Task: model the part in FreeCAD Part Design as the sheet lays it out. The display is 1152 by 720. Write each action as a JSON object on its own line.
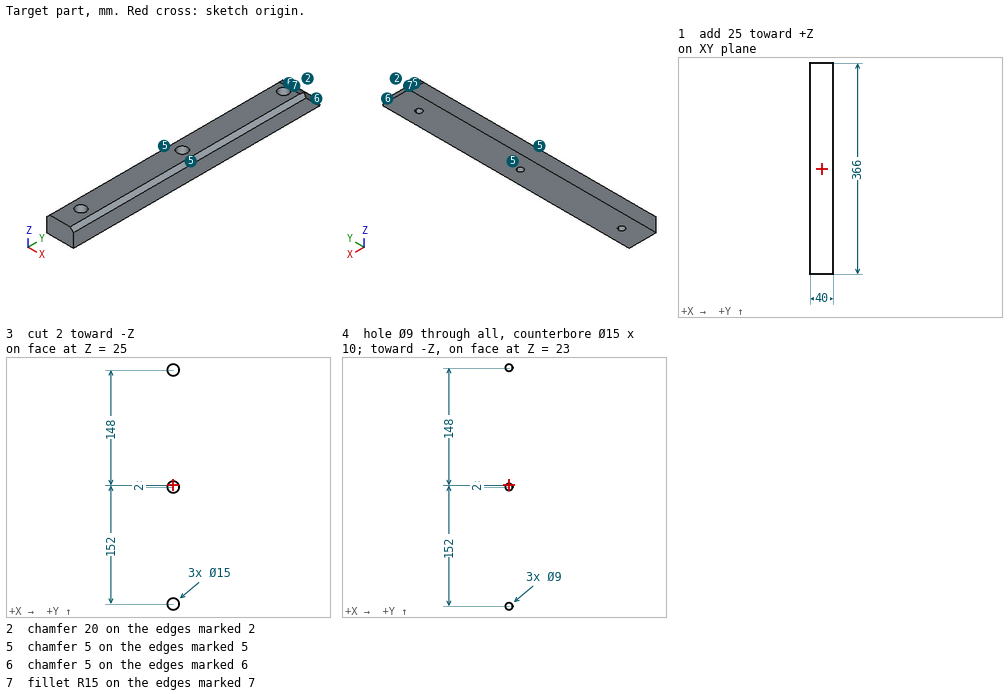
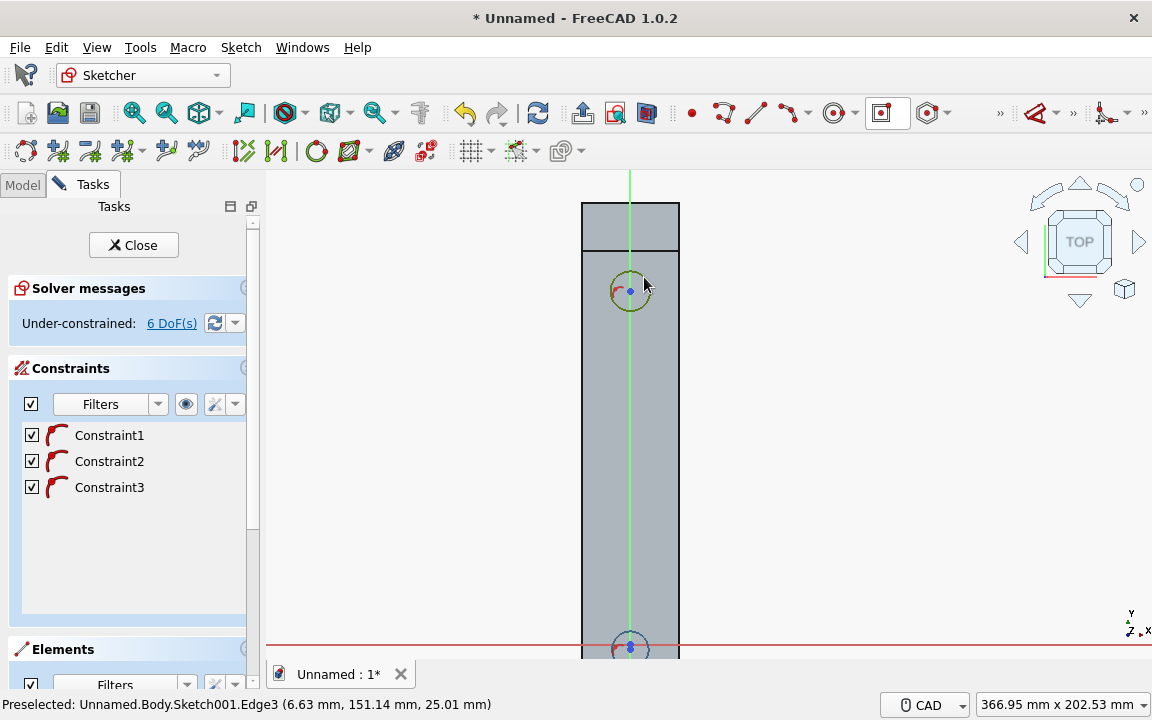
{"action": "key", "text": "e"}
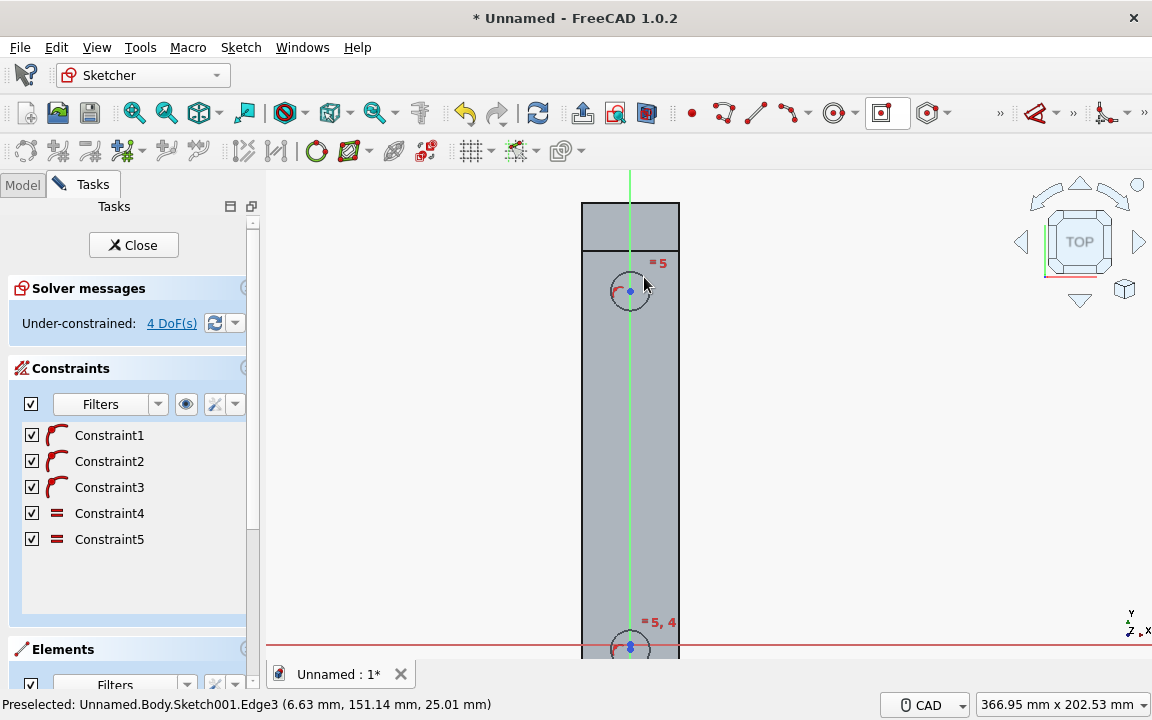
{"action": "left_click", "coordinate": [1036, 114]}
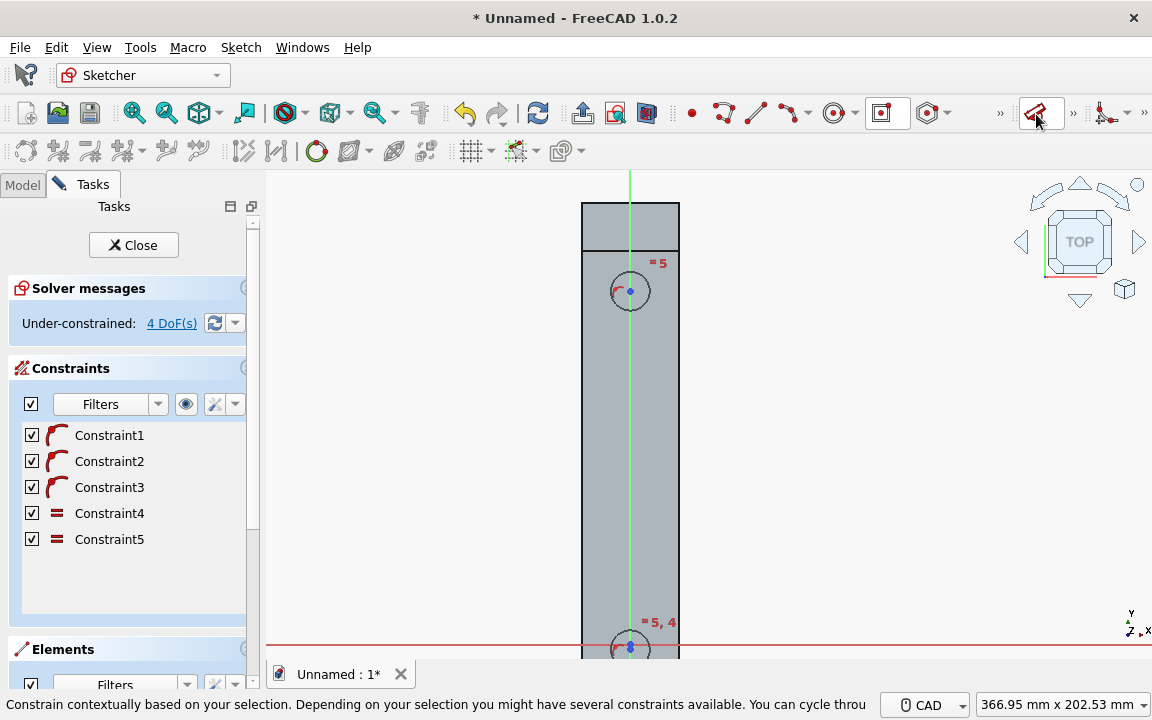
{"action": "scroll", "coordinate": [646, 278], "scroll_direction": "down", "scroll_amount": 5}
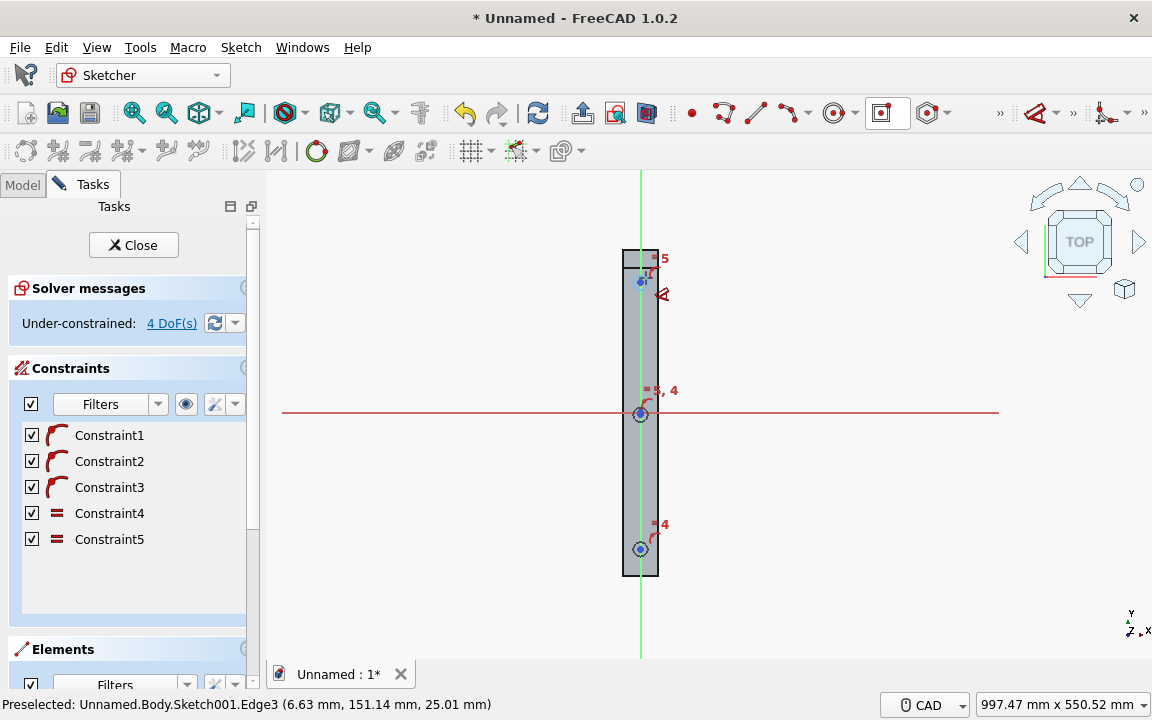
{"action": "scroll", "coordinate": [646, 544], "scroll_direction": "up", "scroll_amount": 6}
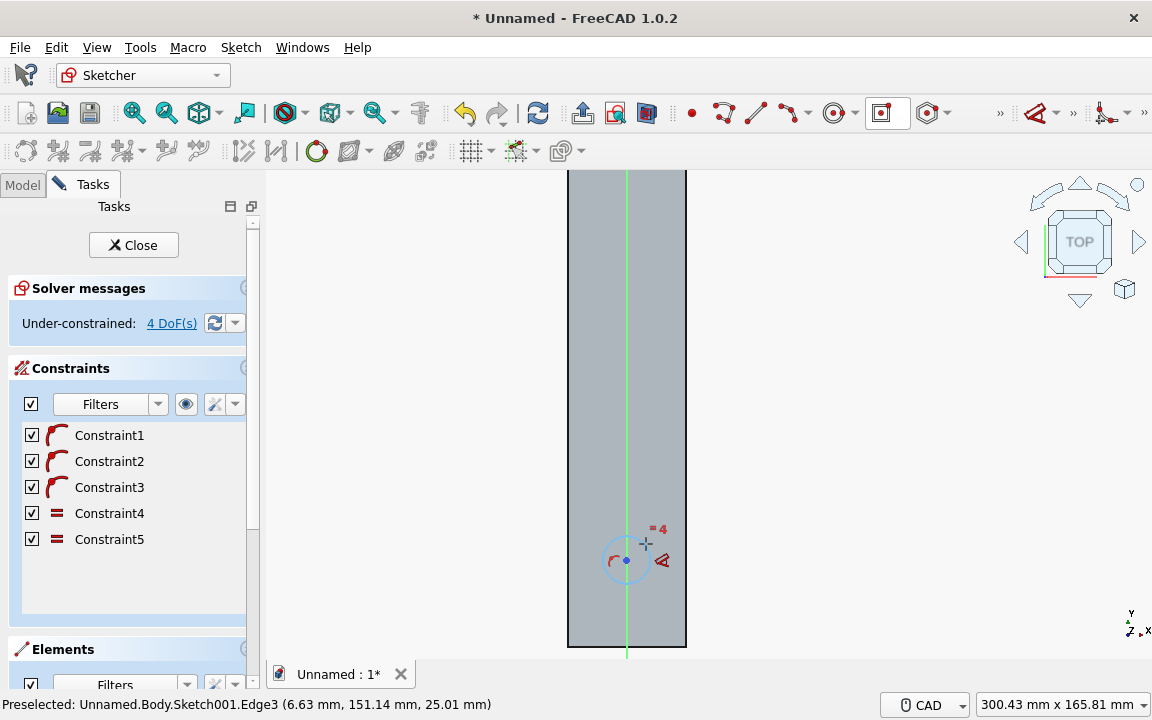
{"action": "left_click", "coordinate": [643, 543]}
{"action": "left_click", "coordinate": [665, 520]}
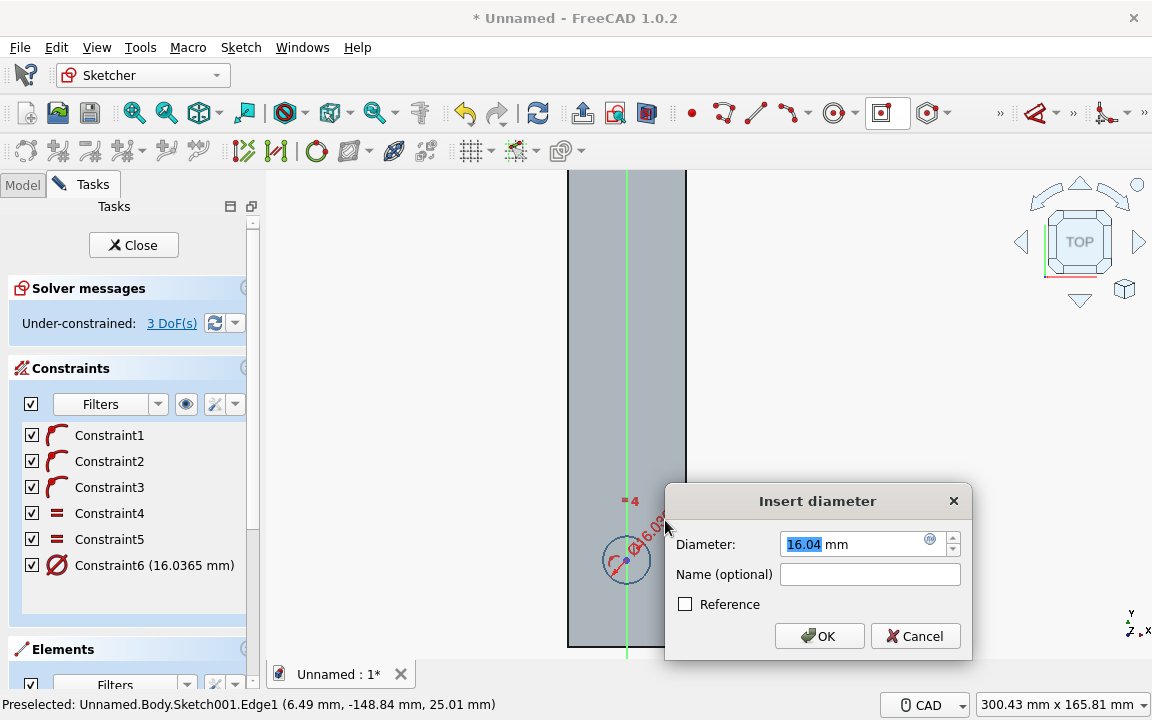
{"action": "type", "text": "15"}
{"action": "key", "text": "Return"}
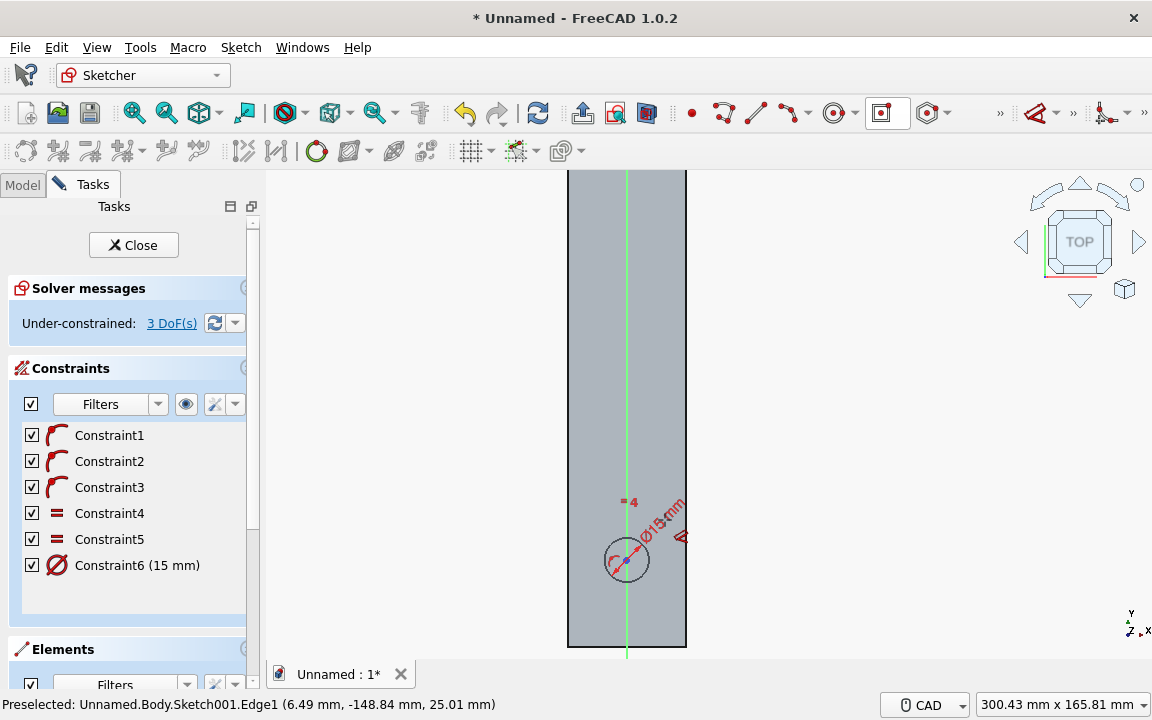
{"action": "scroll", "coordinate": [646, 544], "scroll_direction": "down", "scroll_amount": 6}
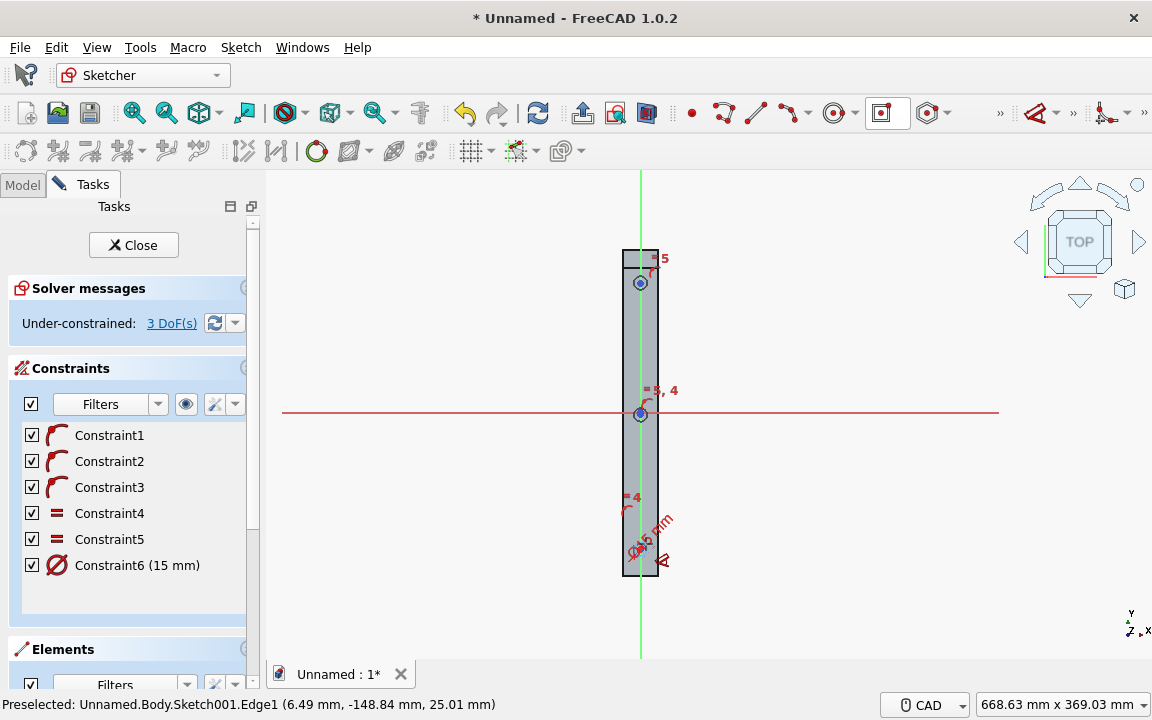
{"action": "scroll", "coordinate": [641, 415], "scroll_direction": "up", "scroll_amount": 16}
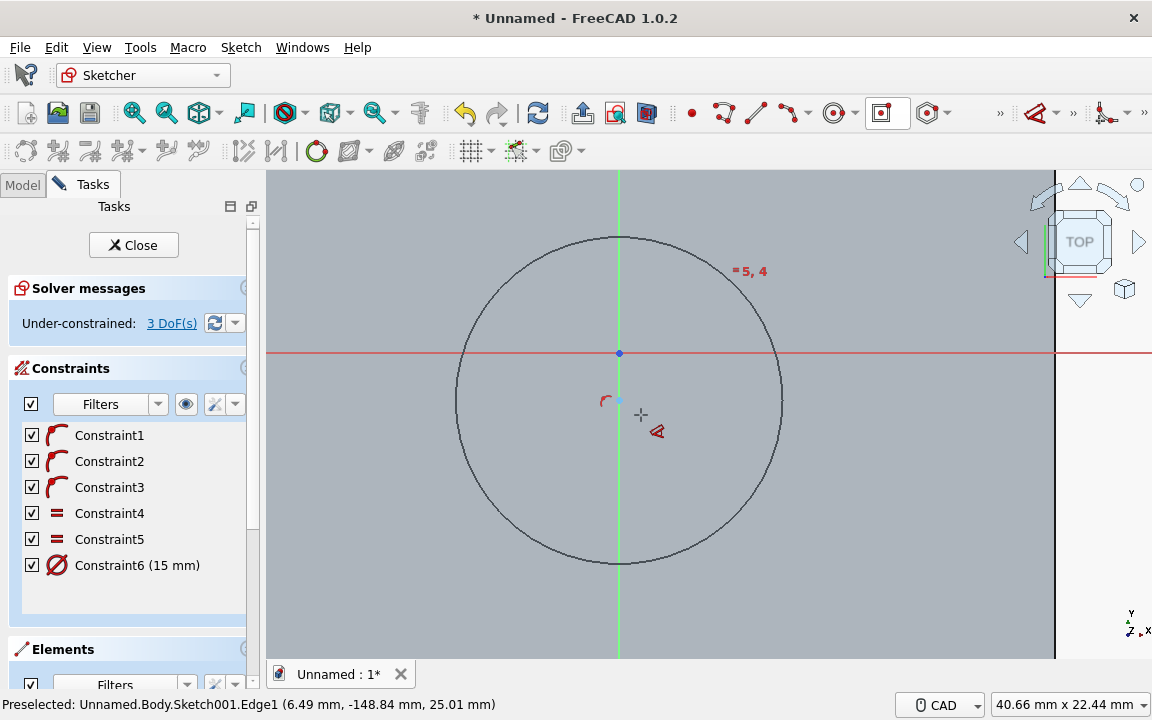
{"action": "left_click", "coordinate": [619, 401]}
{"action": "left_click", "coordinate": [653, 377]}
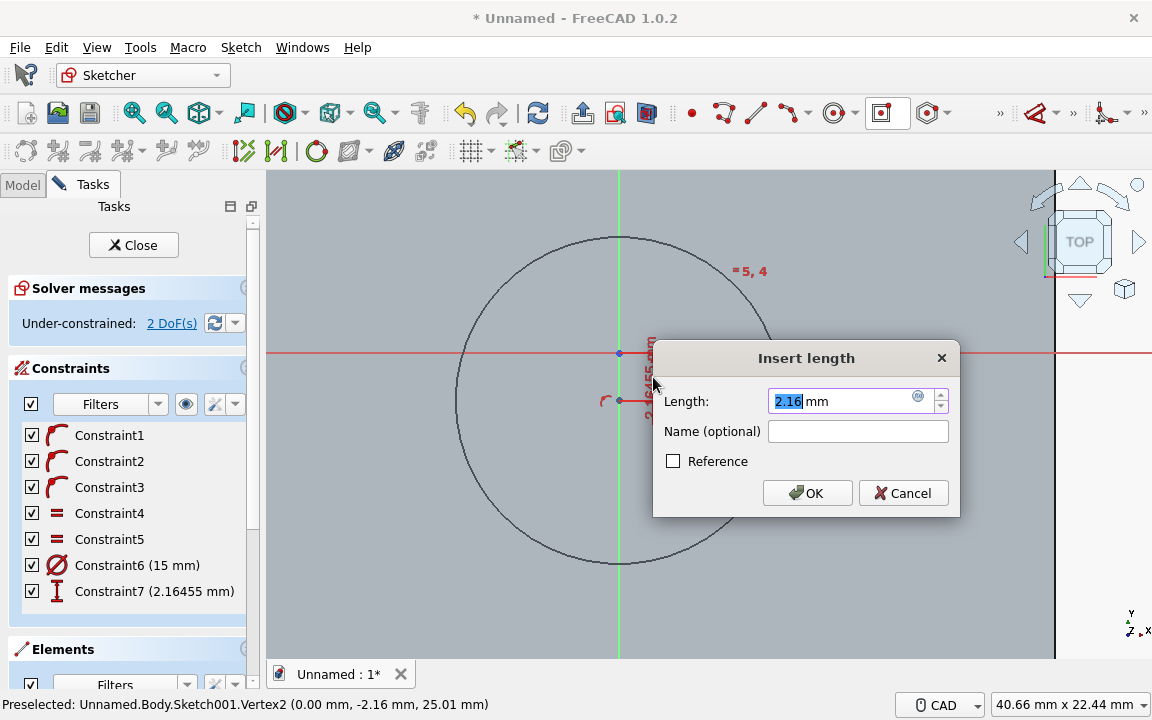
{"action": "type", "text": "2"}
{"action": "key", "text": "Return"}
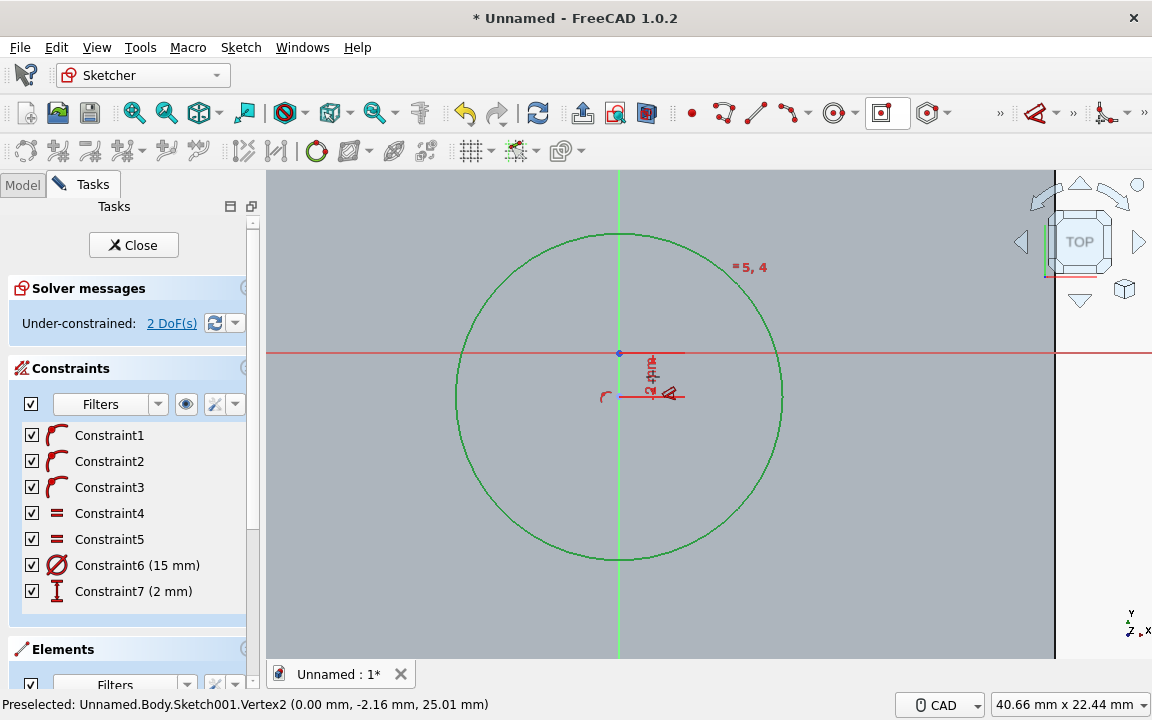
{"action": "scroll", "coordinate": [642, 415], "scroll_direction": "down", "scroll_amount": 15}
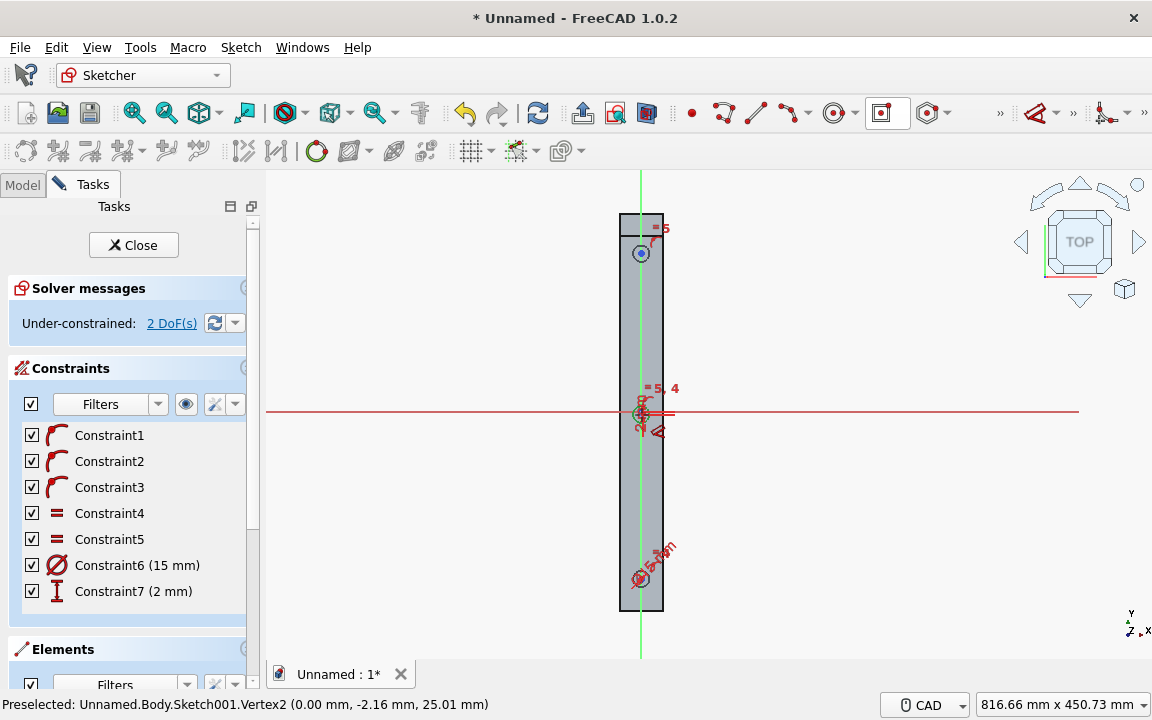
{"action": "left_click", "coordinate": [641, 579]}
{"action": "left_click", "coordinate": [675, 496]}